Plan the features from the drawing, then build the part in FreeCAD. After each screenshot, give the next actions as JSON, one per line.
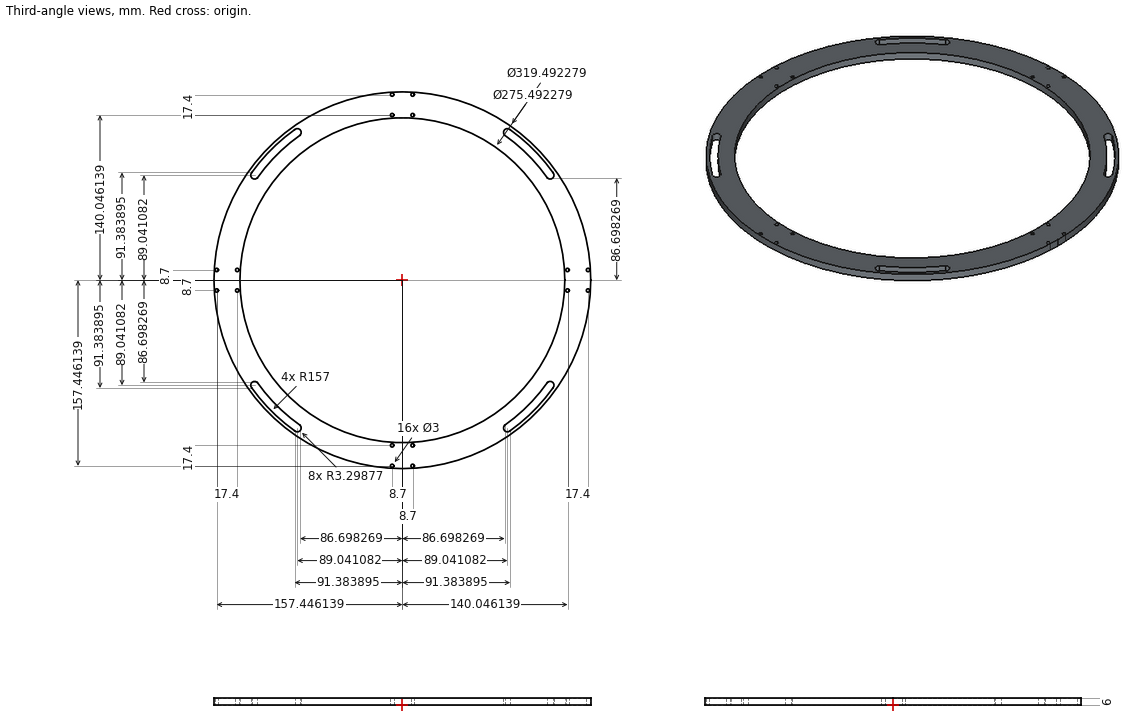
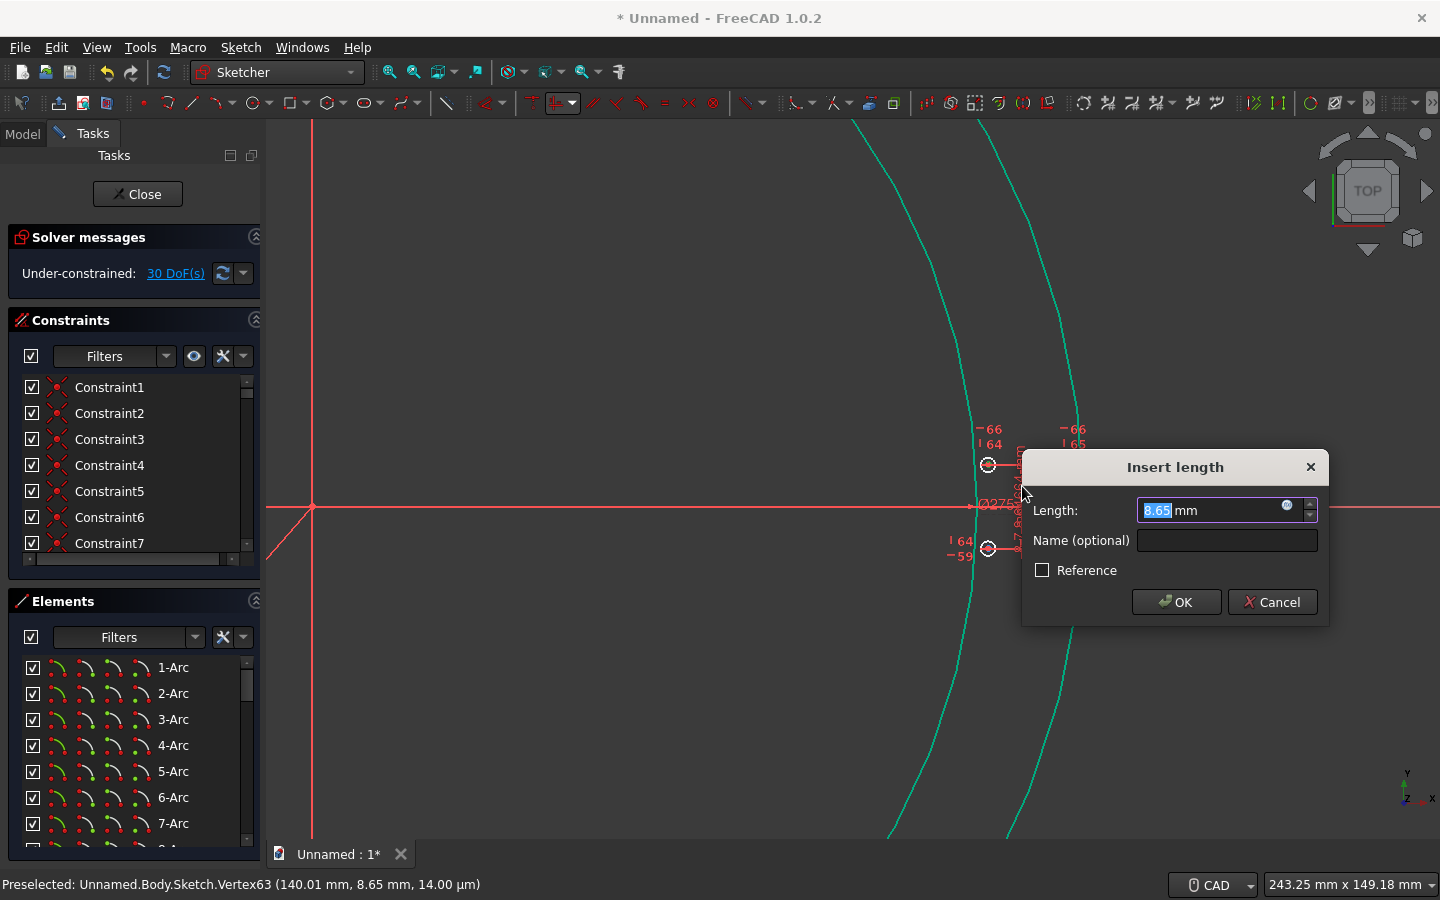
{"action": "type", "text": "8.7"}
{"action": "key", "text": "Return"}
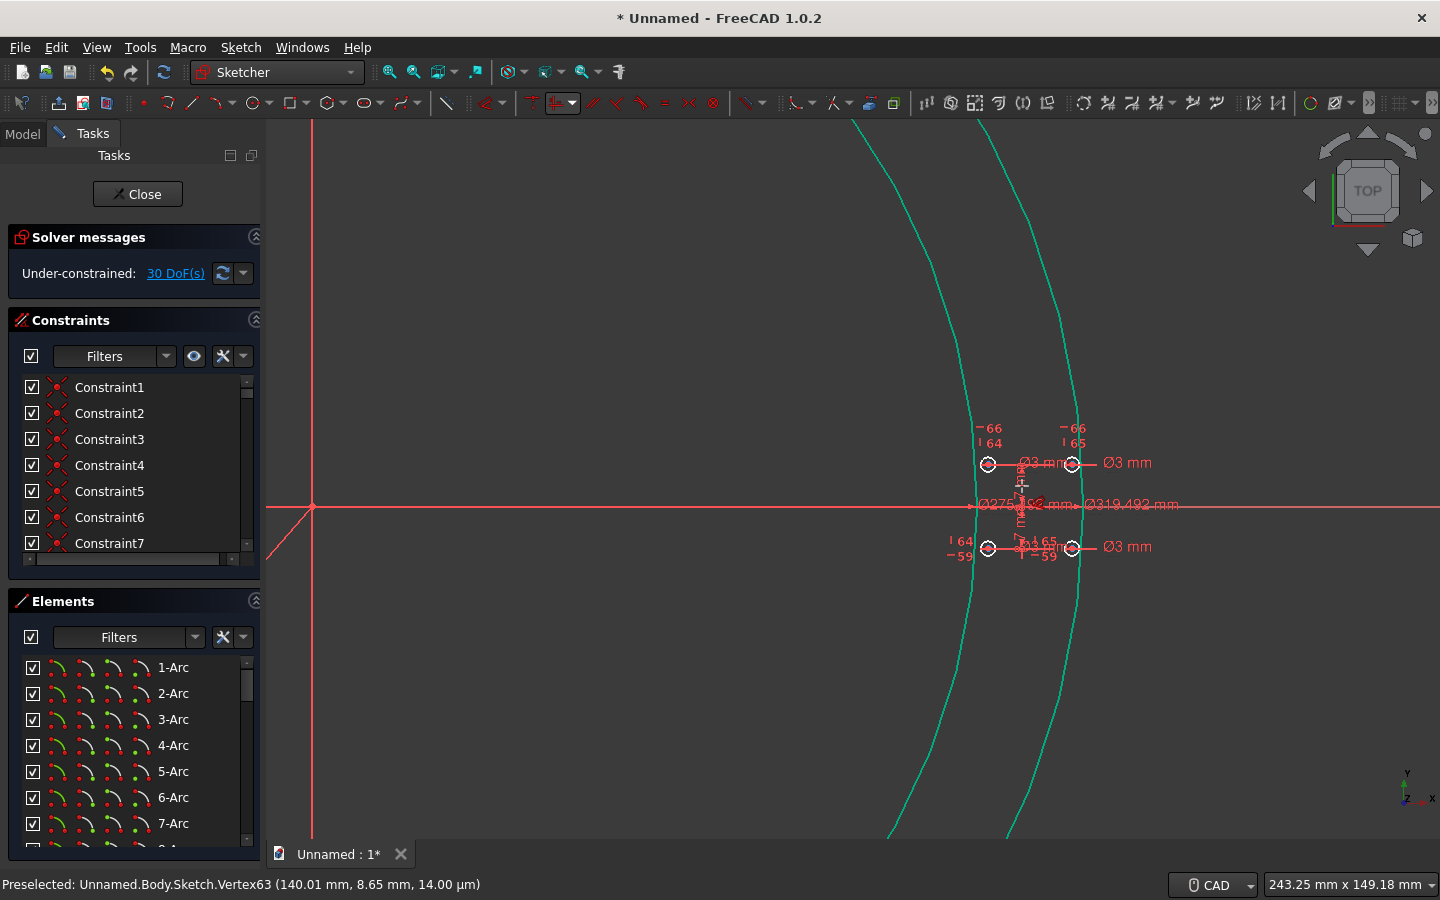
{"action": "scroll", "coordinate": [988, 467], "scroll_direction": "down", "scroll_amount": 6}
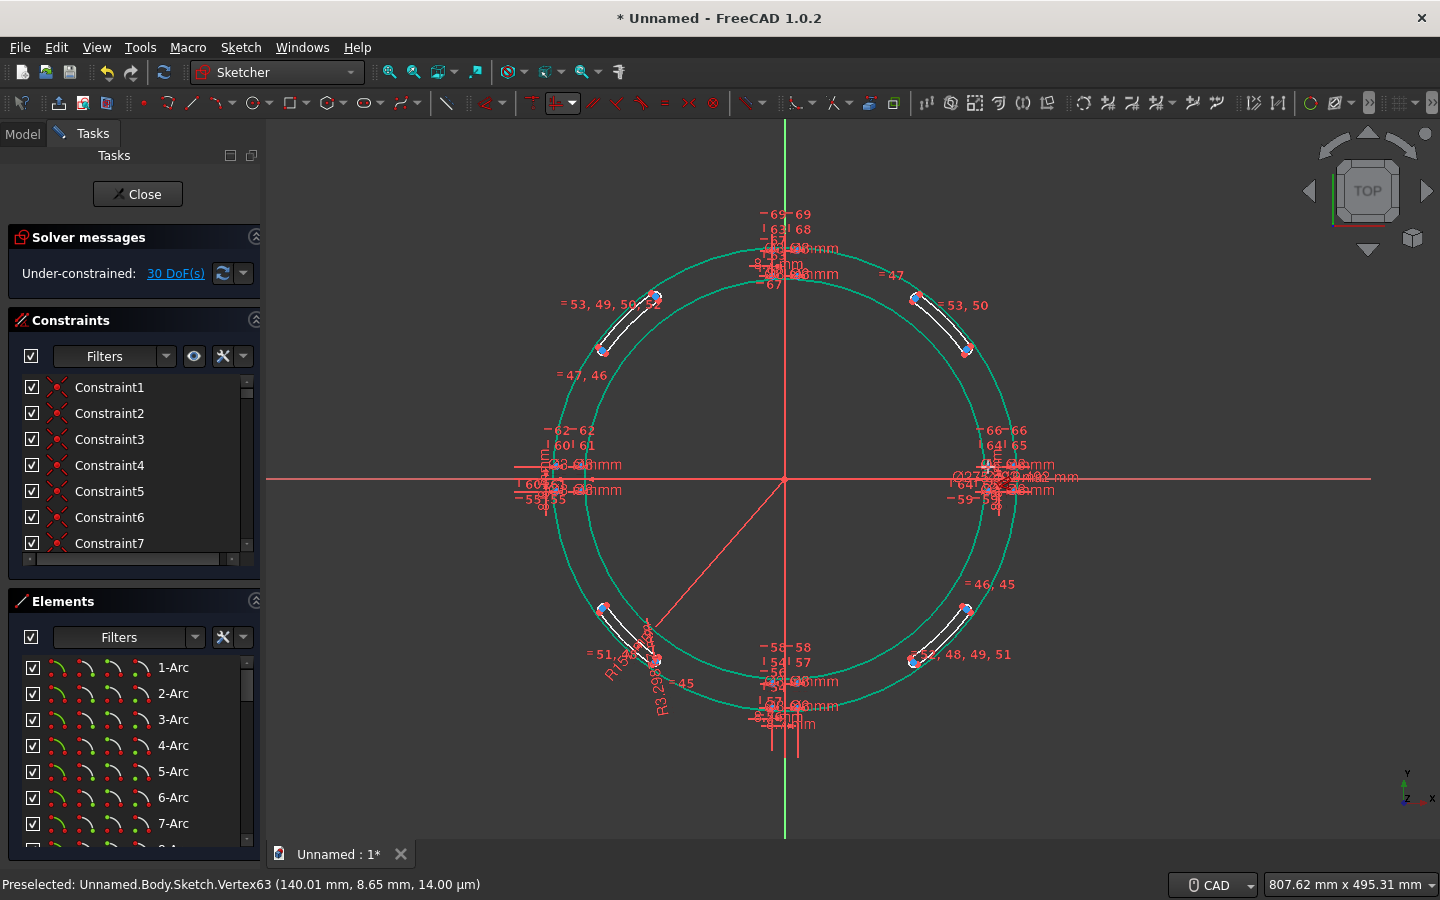
{"action": "scroll", "coordinate": [798, 276], "scroll_direction": "up", "scroll_amount": 6}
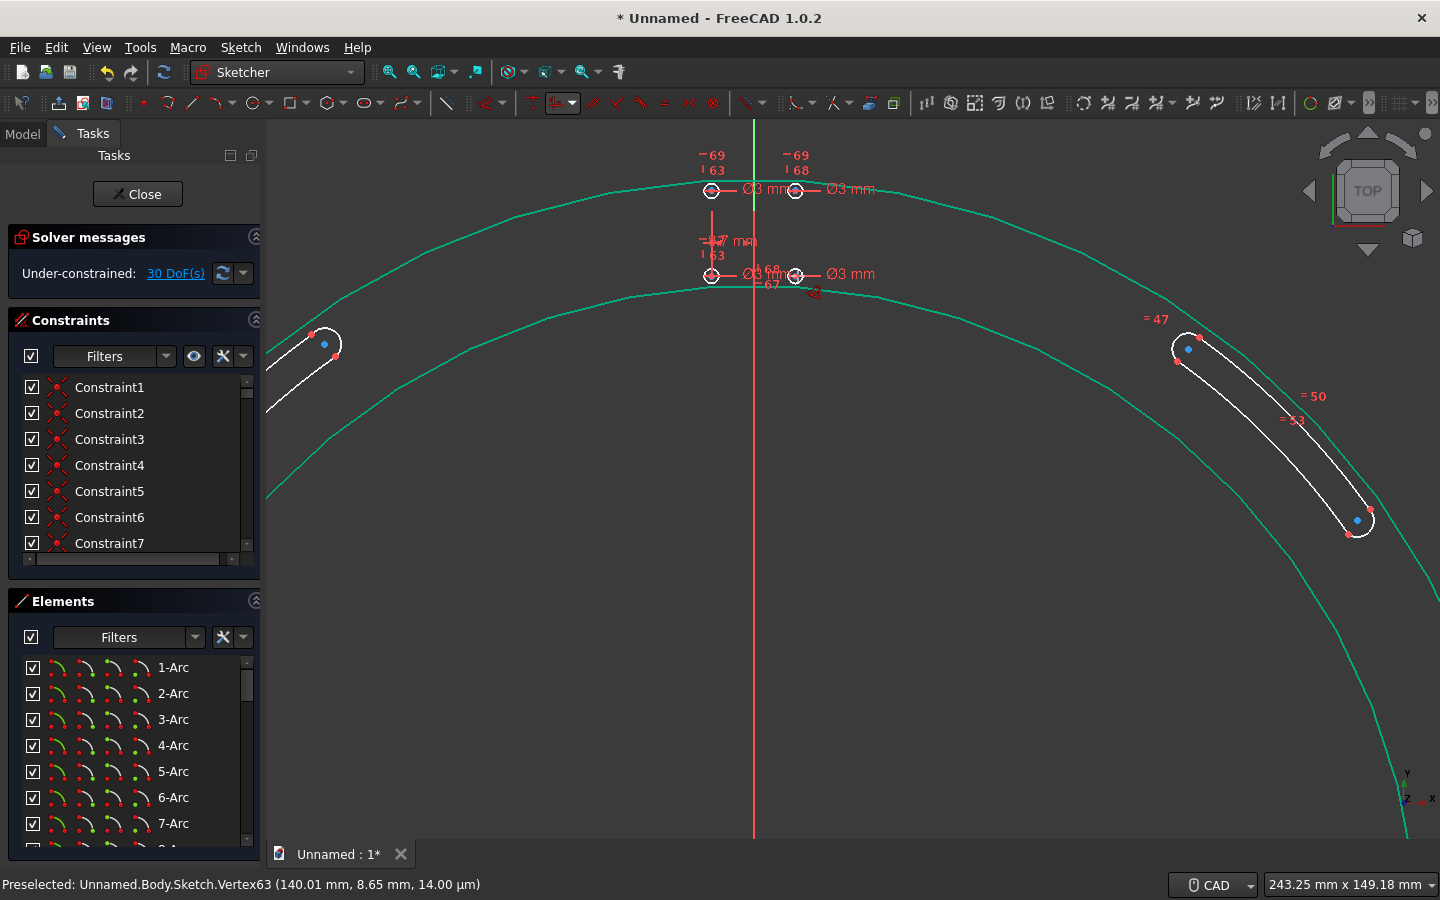
{"action": "left_click", "coordinate": [795, 276]}
{"action": "left_click", "coordinate": [774, 218]}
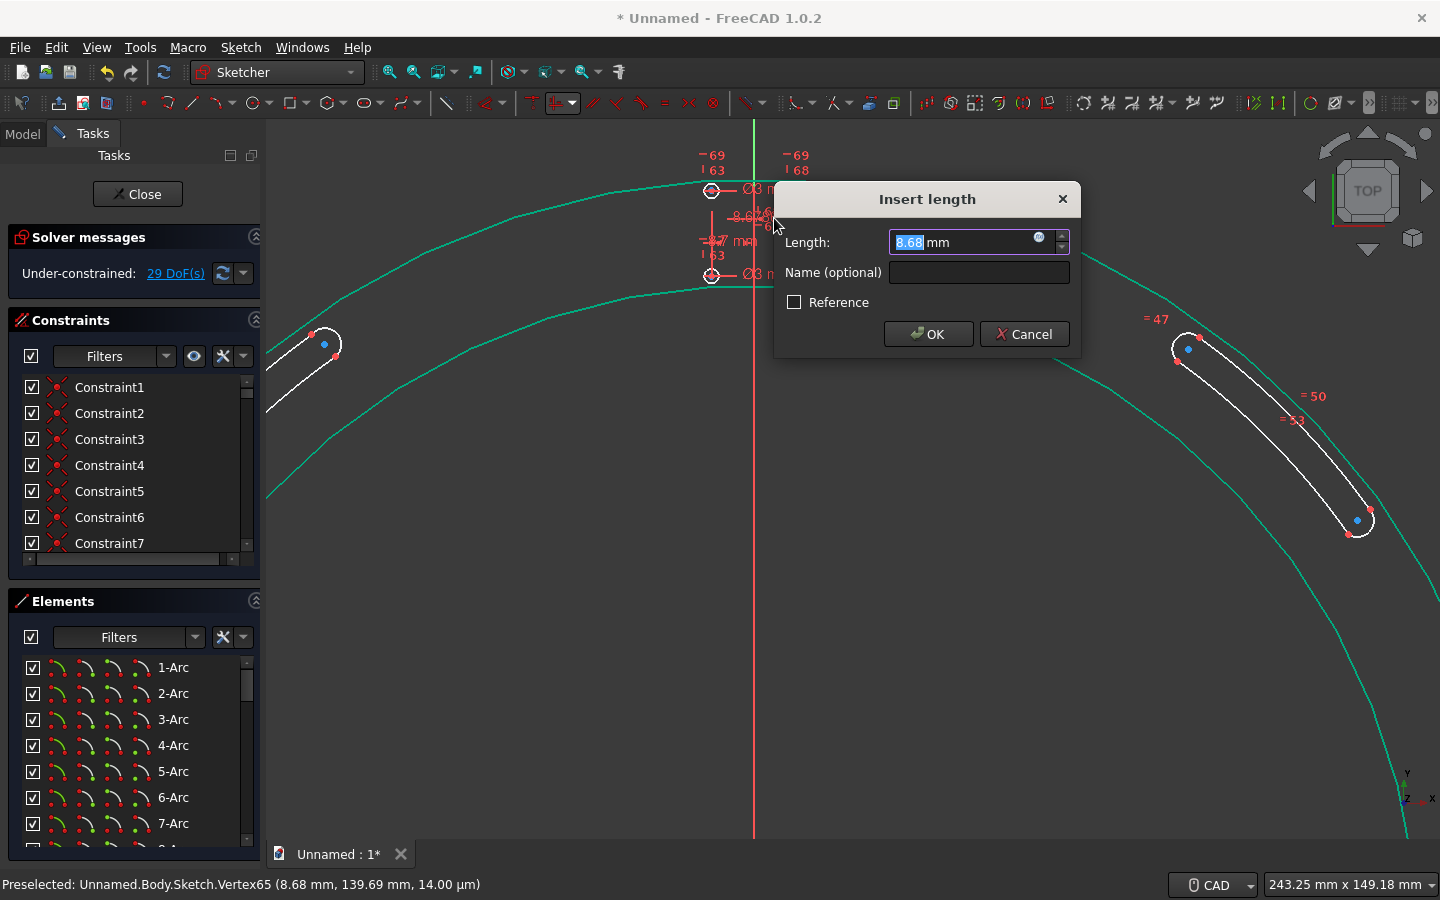
{"action": "type", "text": "8.7"}
{"action": "key", "text": "Return"}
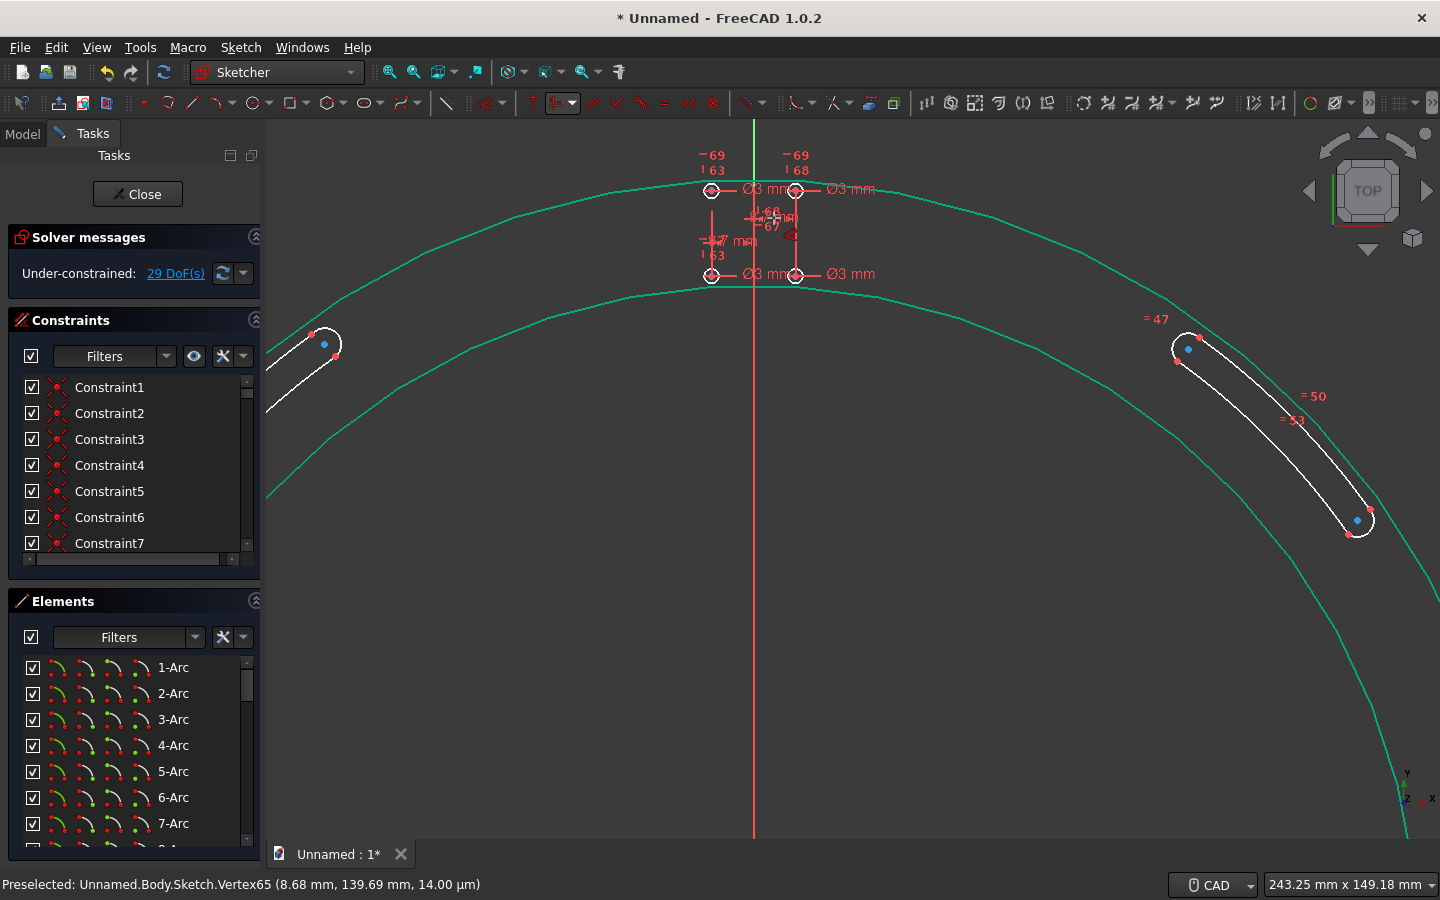
{"action": "scroll", "coordinate": [798, 276], "scroll_direction": "down", "scroll_amount": 6}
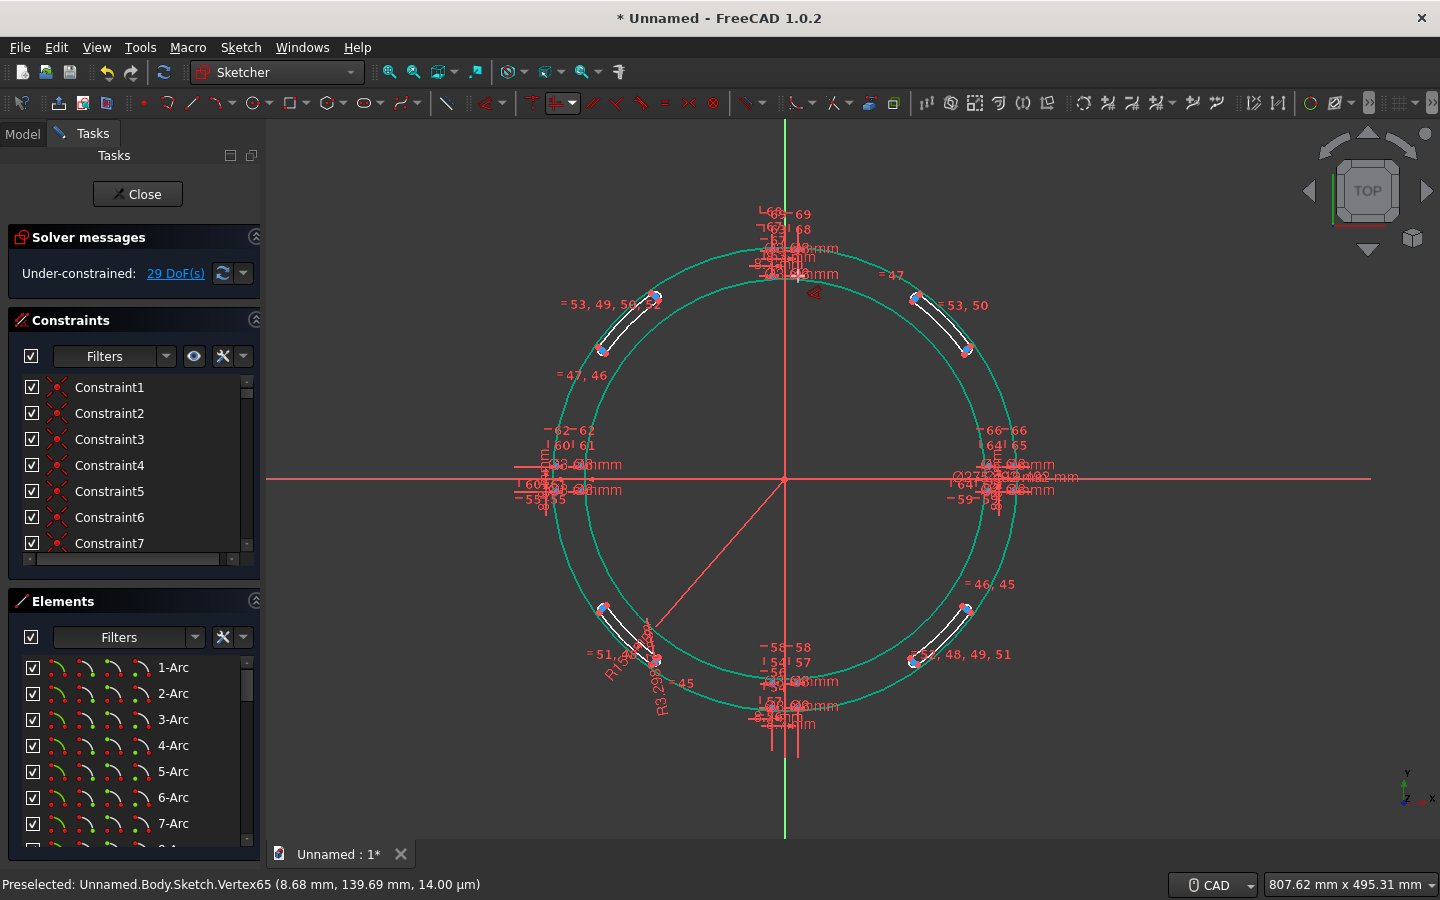
{"action": "scroll", "coordinate": [772, 708], "scroll_direction": "up", "scroll_amount": 3}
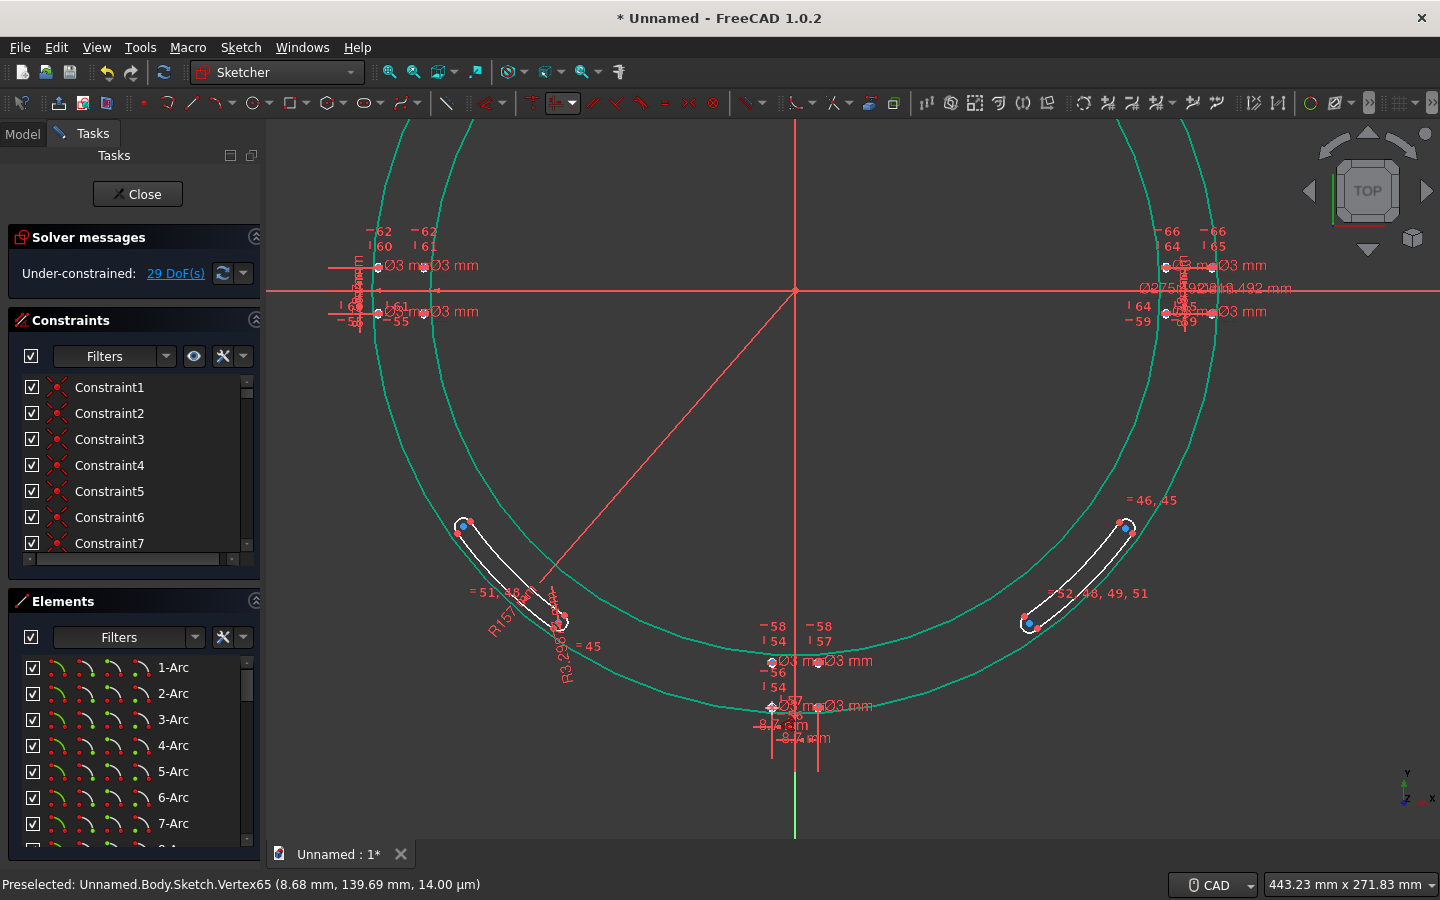
{"action": "left_click", "coordinate": [772, 708]}